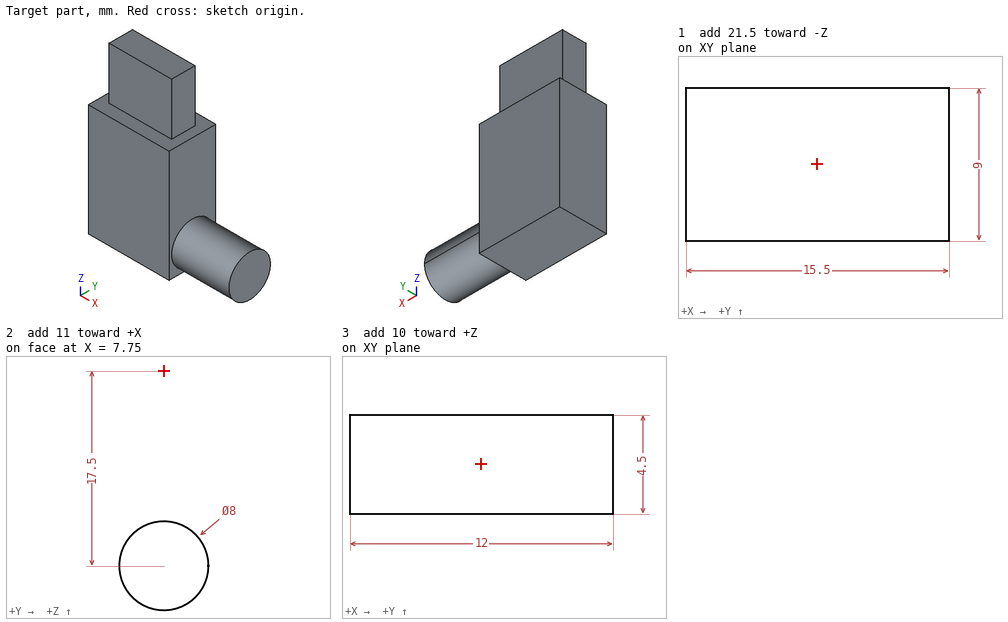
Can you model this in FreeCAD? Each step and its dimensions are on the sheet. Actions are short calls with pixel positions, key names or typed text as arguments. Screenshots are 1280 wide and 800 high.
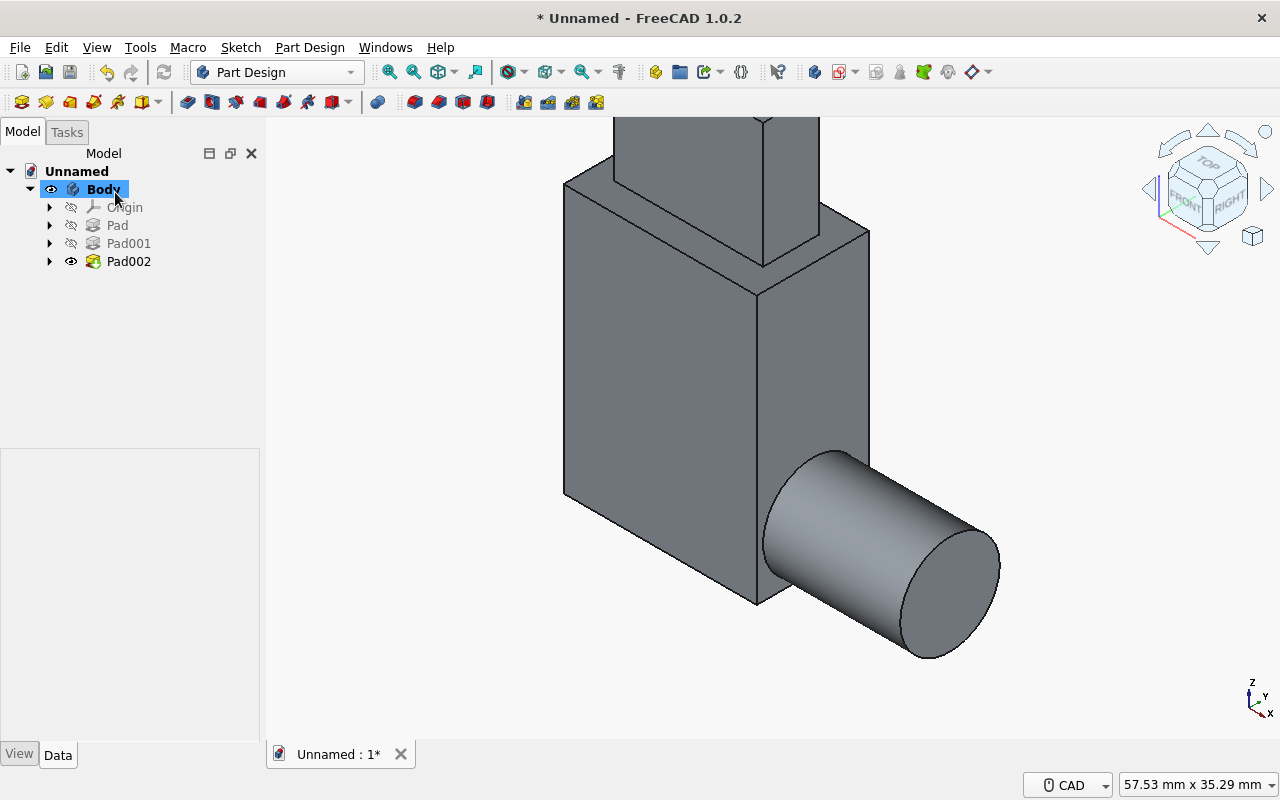
click(390, 72)